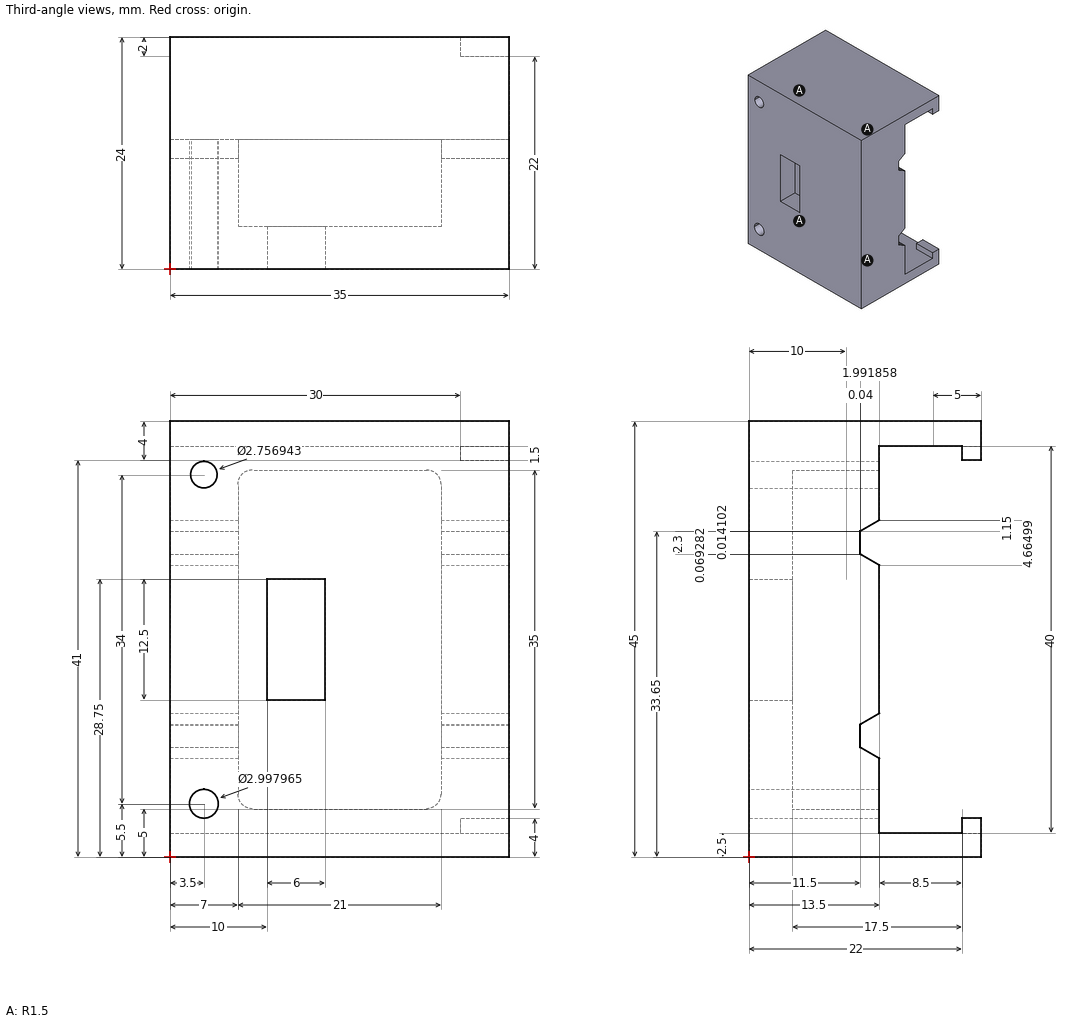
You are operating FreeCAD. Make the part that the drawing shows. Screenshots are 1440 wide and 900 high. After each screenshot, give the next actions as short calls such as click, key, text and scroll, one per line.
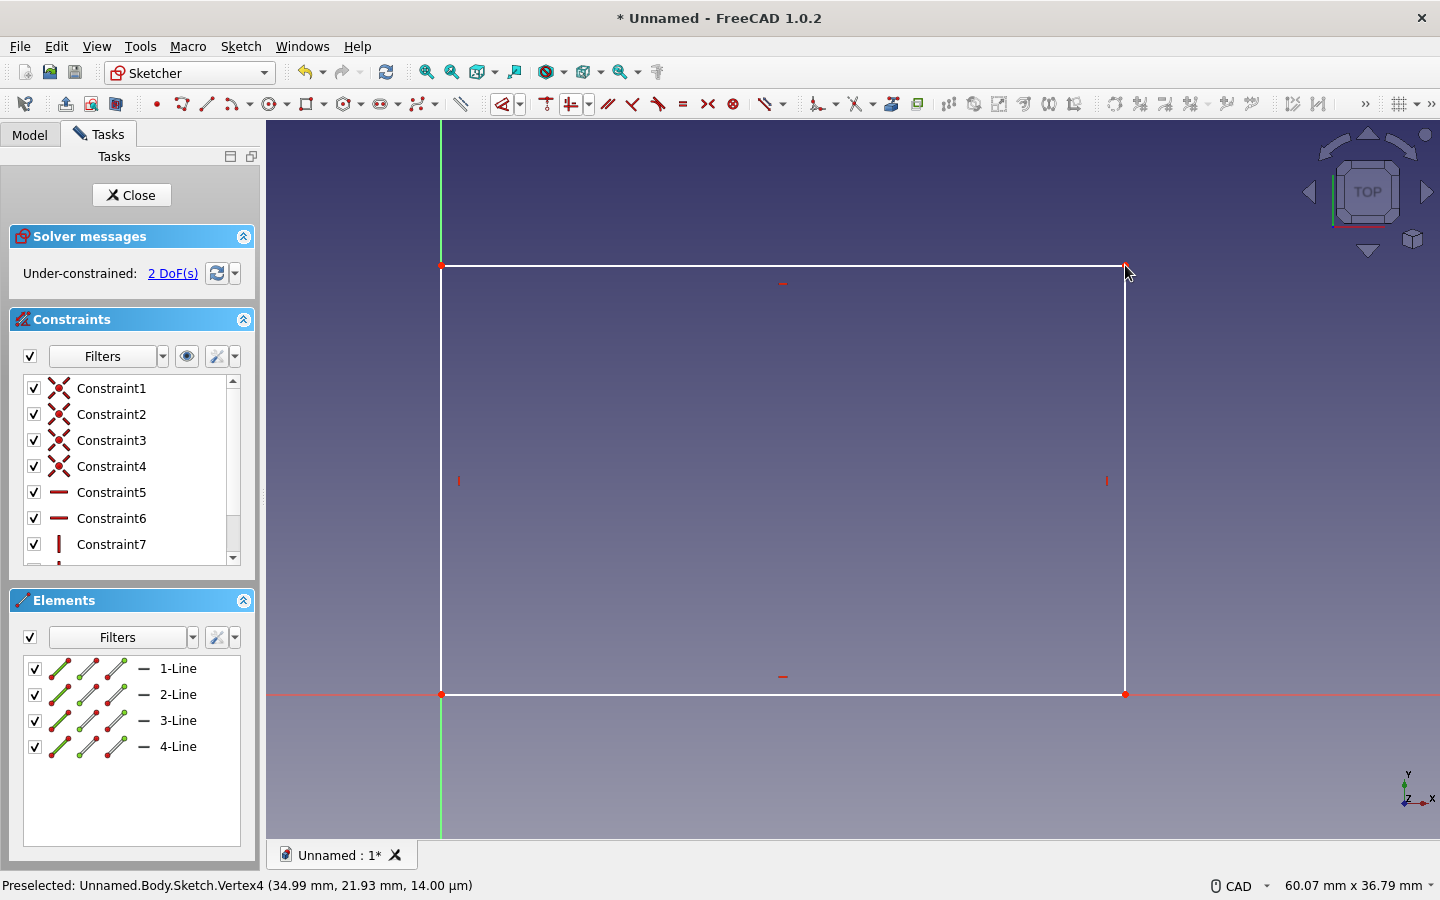
click(502, 104)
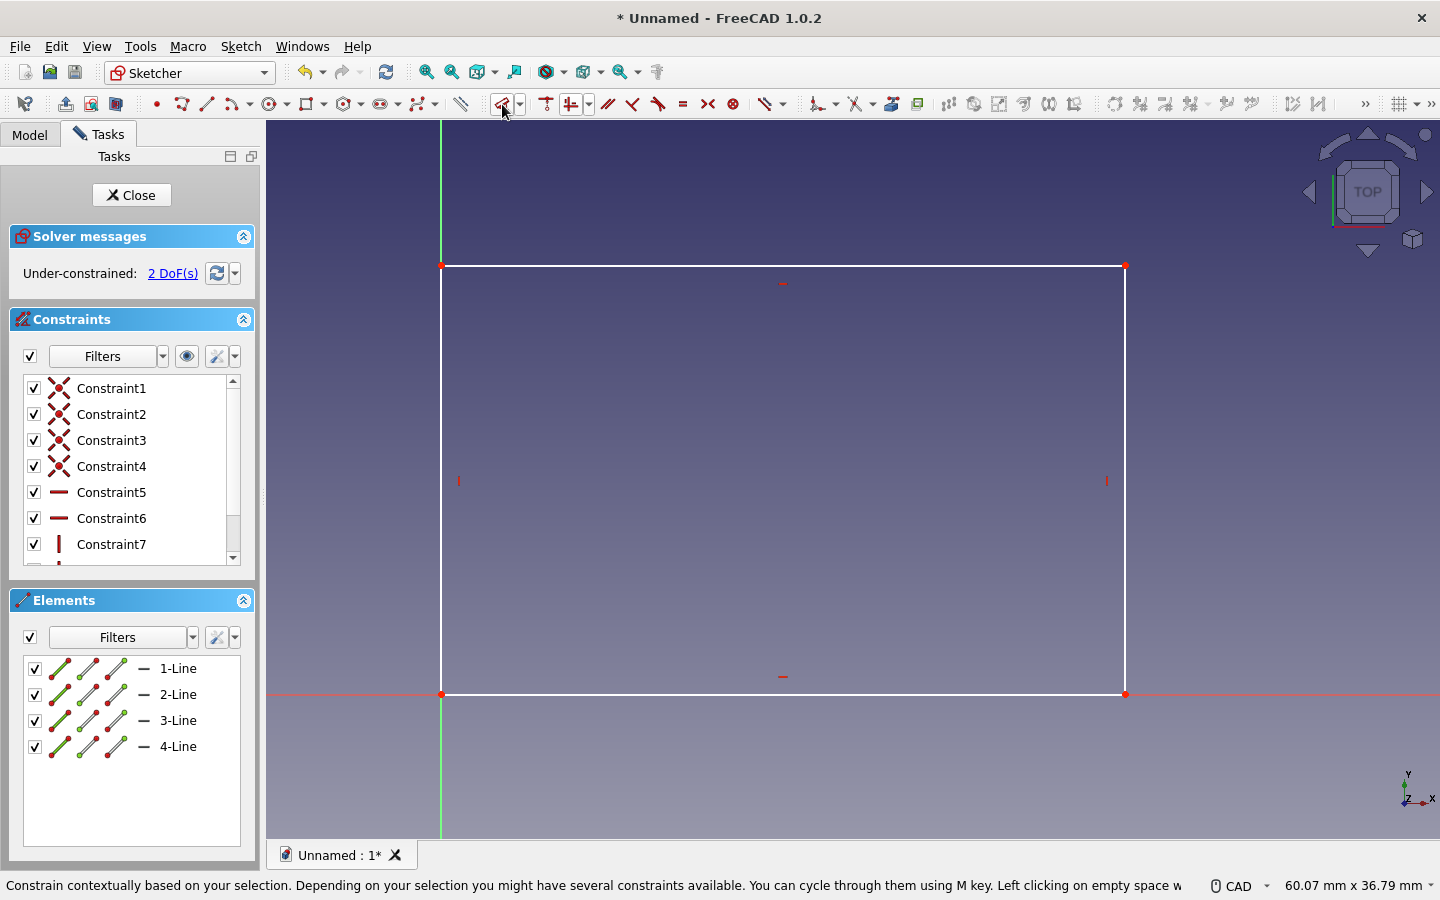
click(646, 695)
click(783, 729)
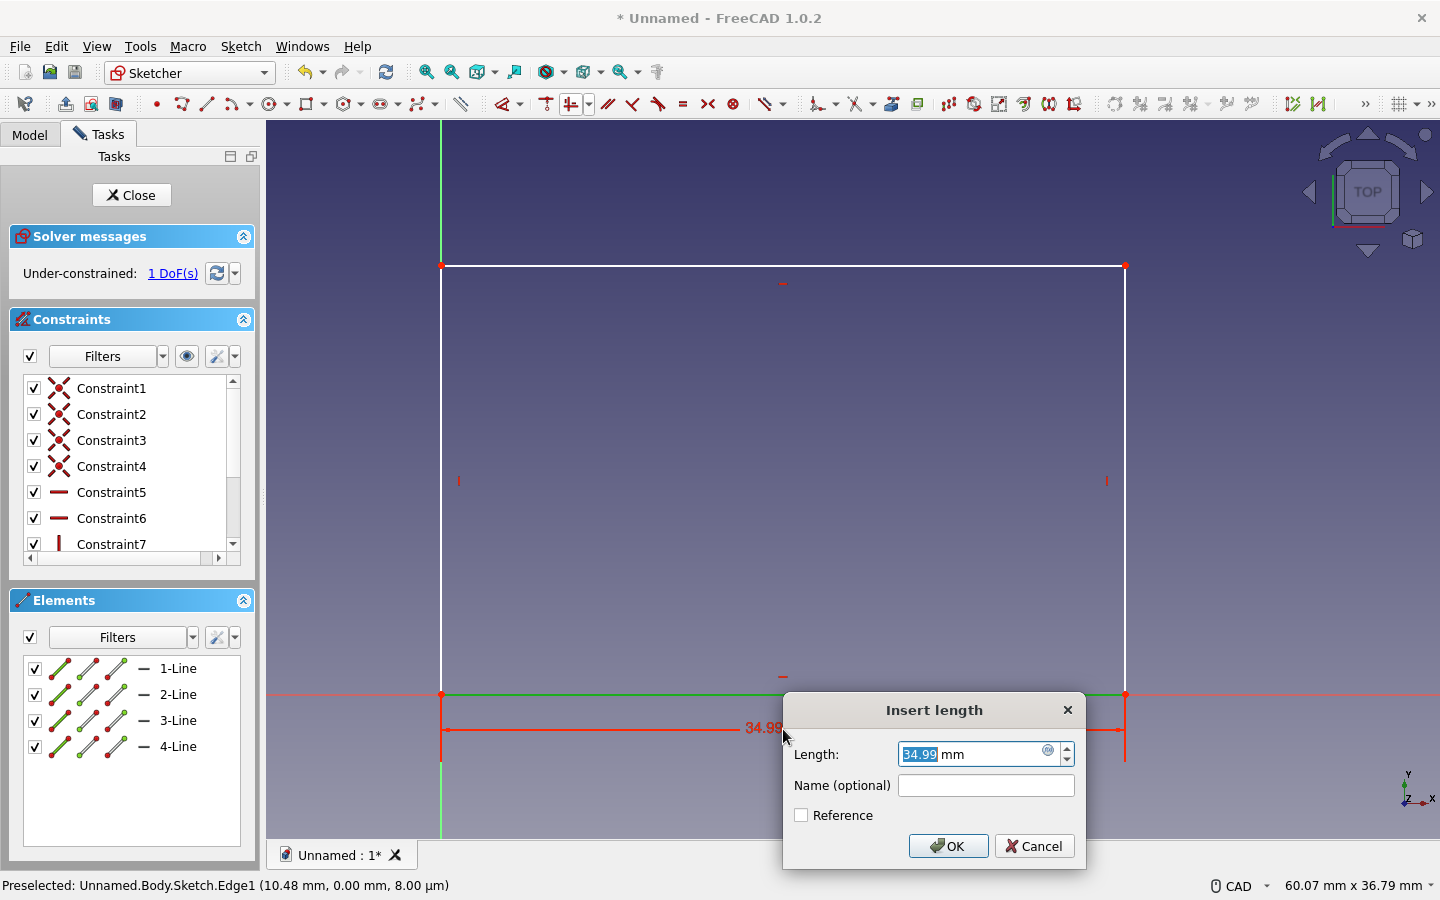
text(35)
key(Return)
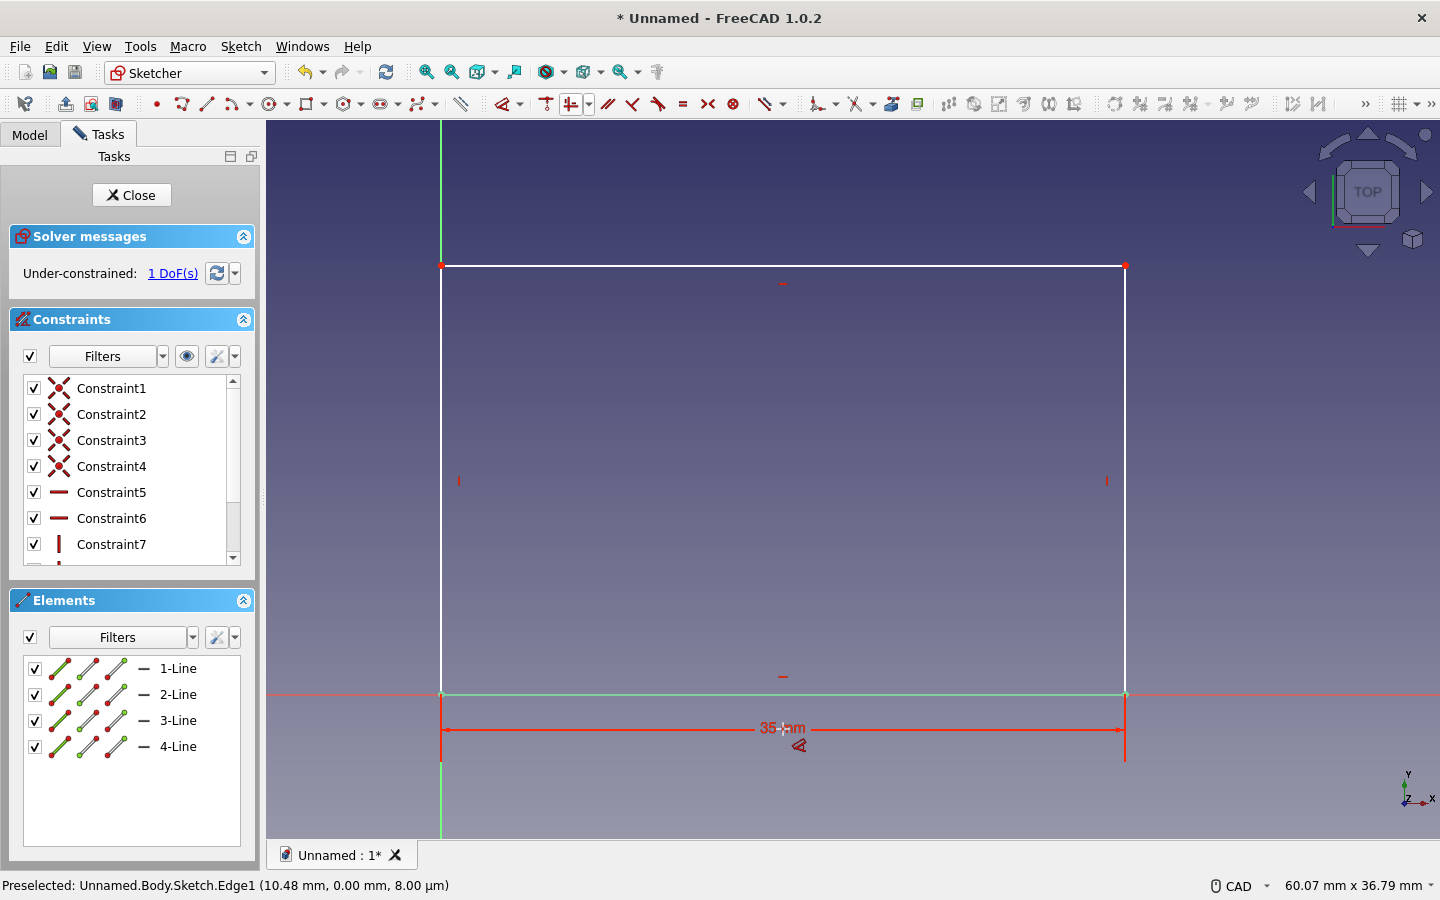
click(1125, 566)
click(1159, 480)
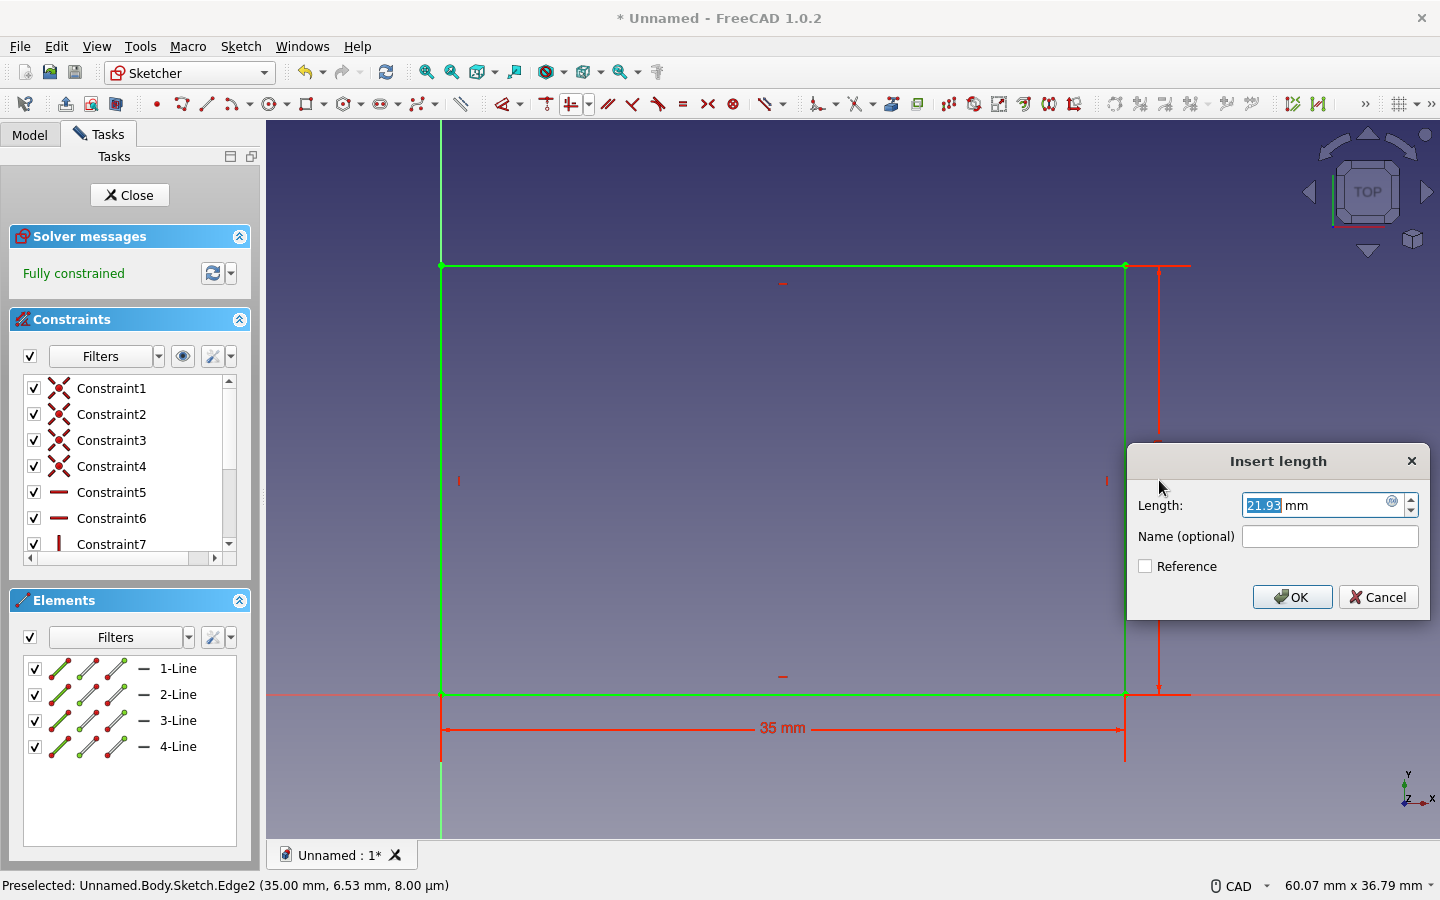
text(22)
key(Return)
key(Escape)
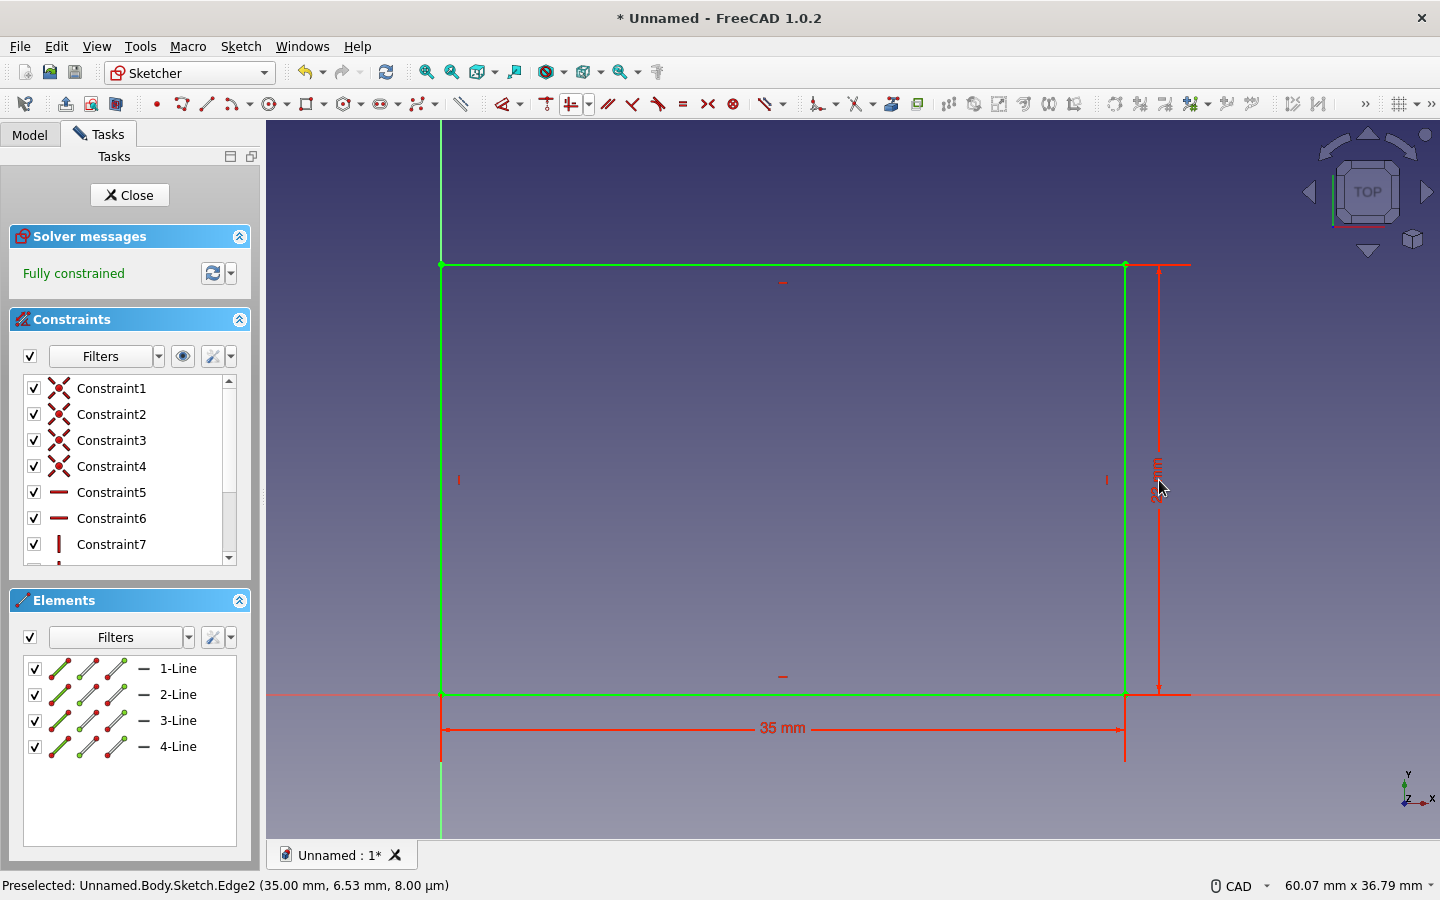
click(130, 195)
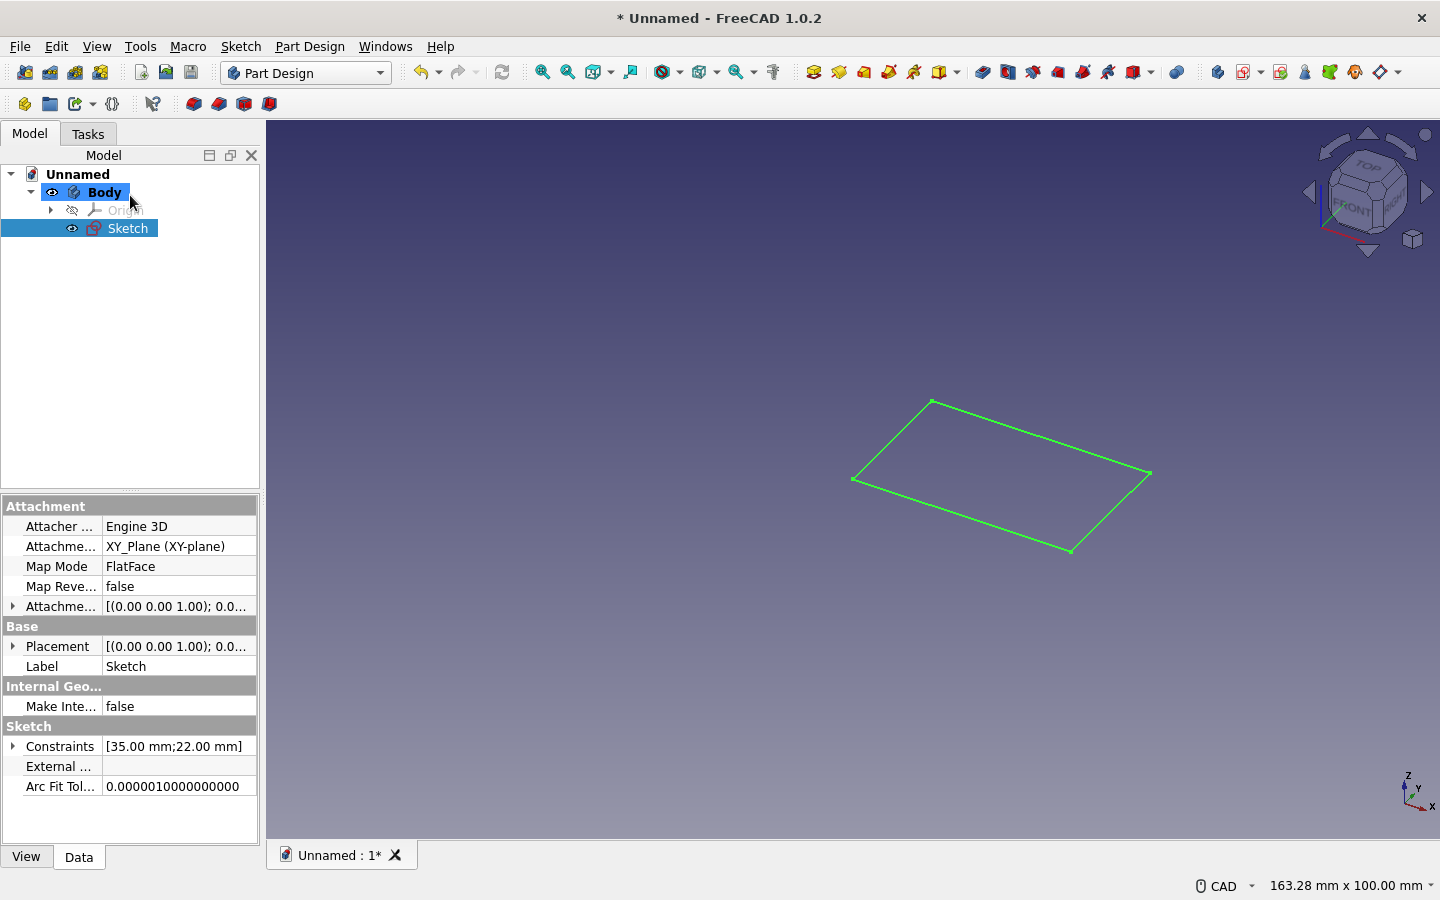
click(814, 72)